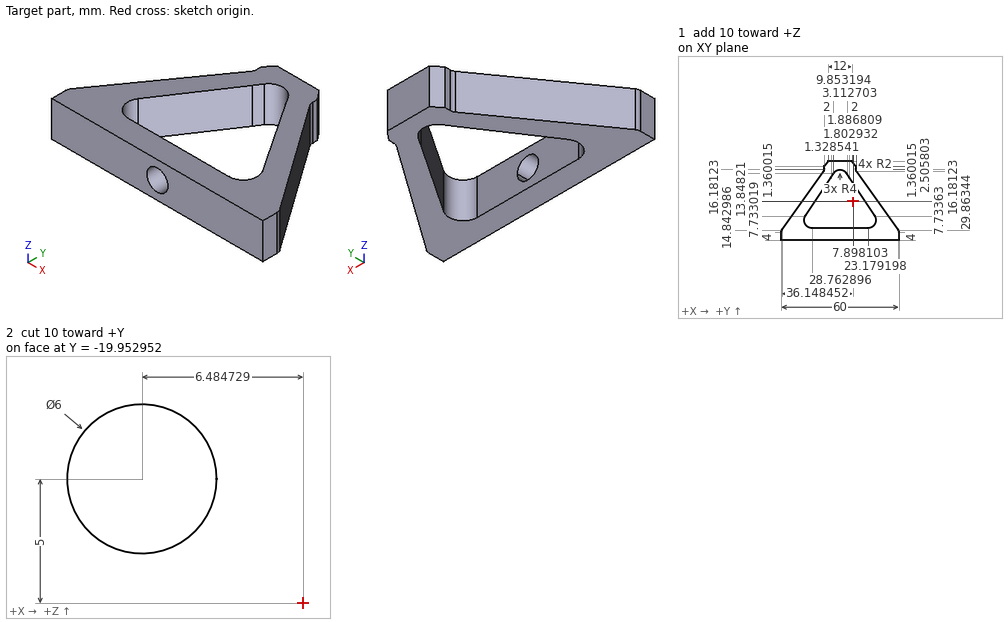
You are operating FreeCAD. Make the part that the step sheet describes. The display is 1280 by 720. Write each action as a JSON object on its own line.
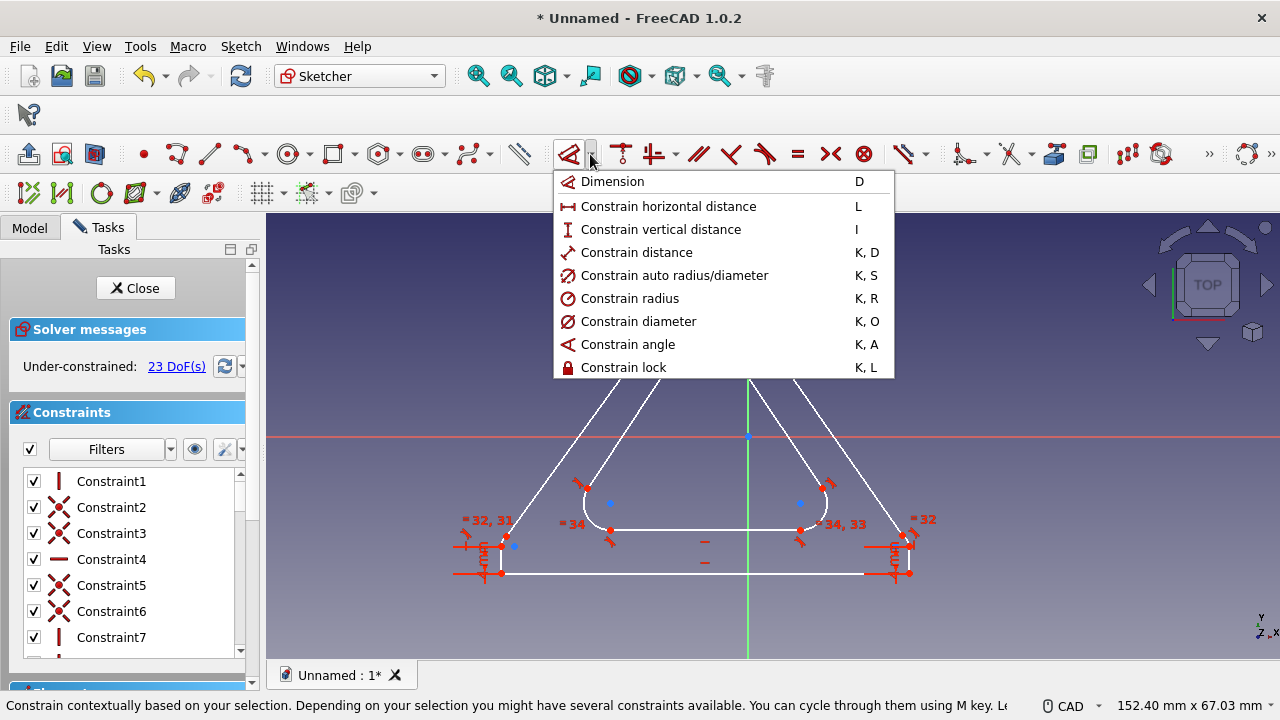
{"action": "left_click", "coordinate": [724, 206]}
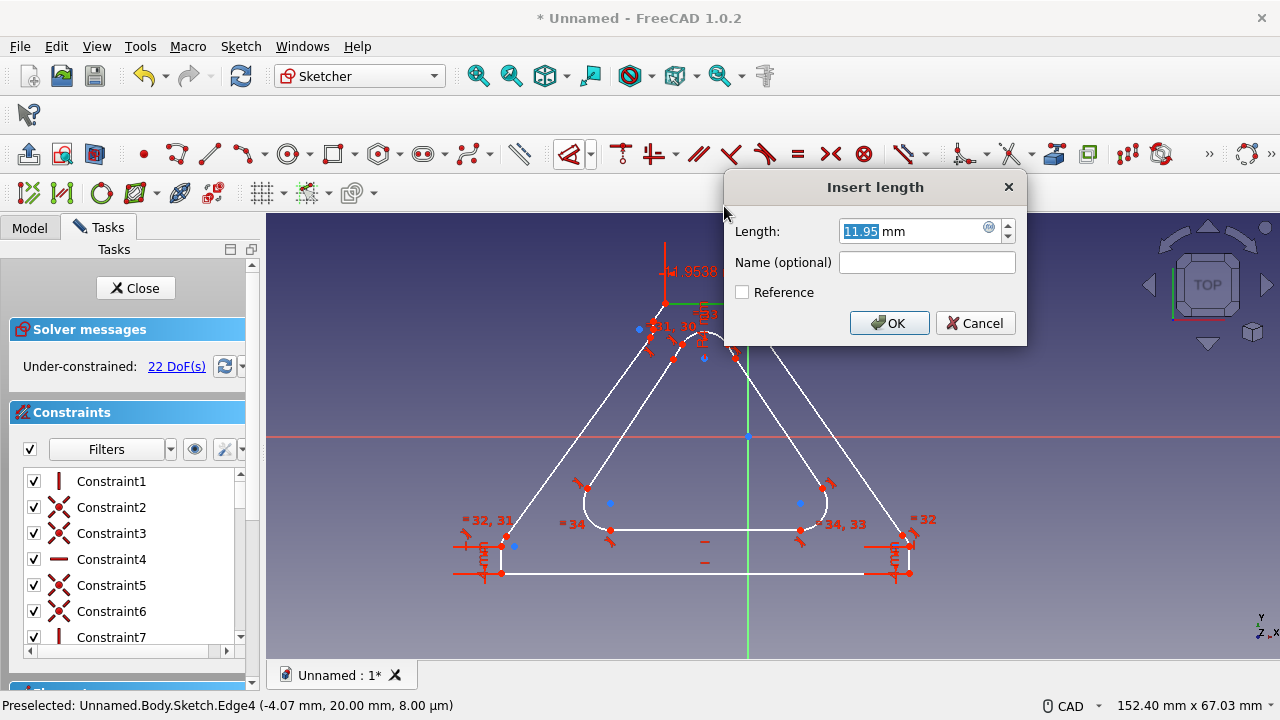
{"action": "type", "text": "12"}
{"action": "key", "text": "Return"}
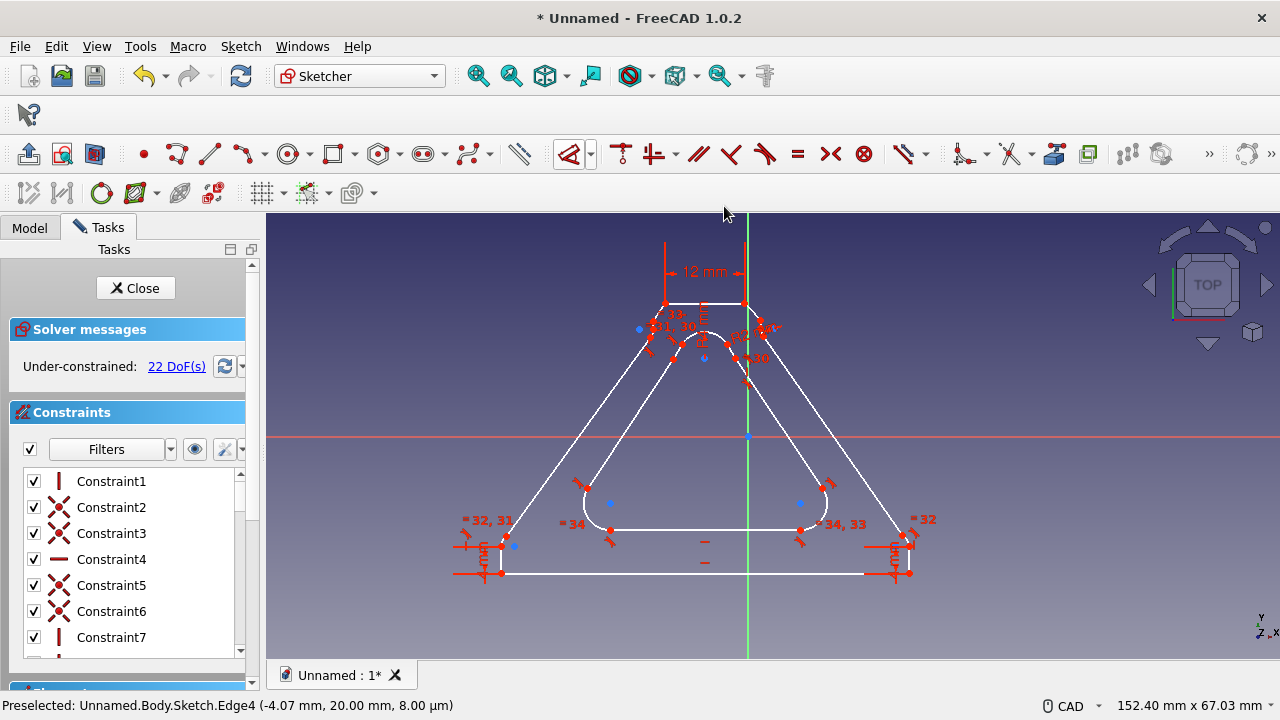
{"action": "left_click", "coordinate": [624, 574]}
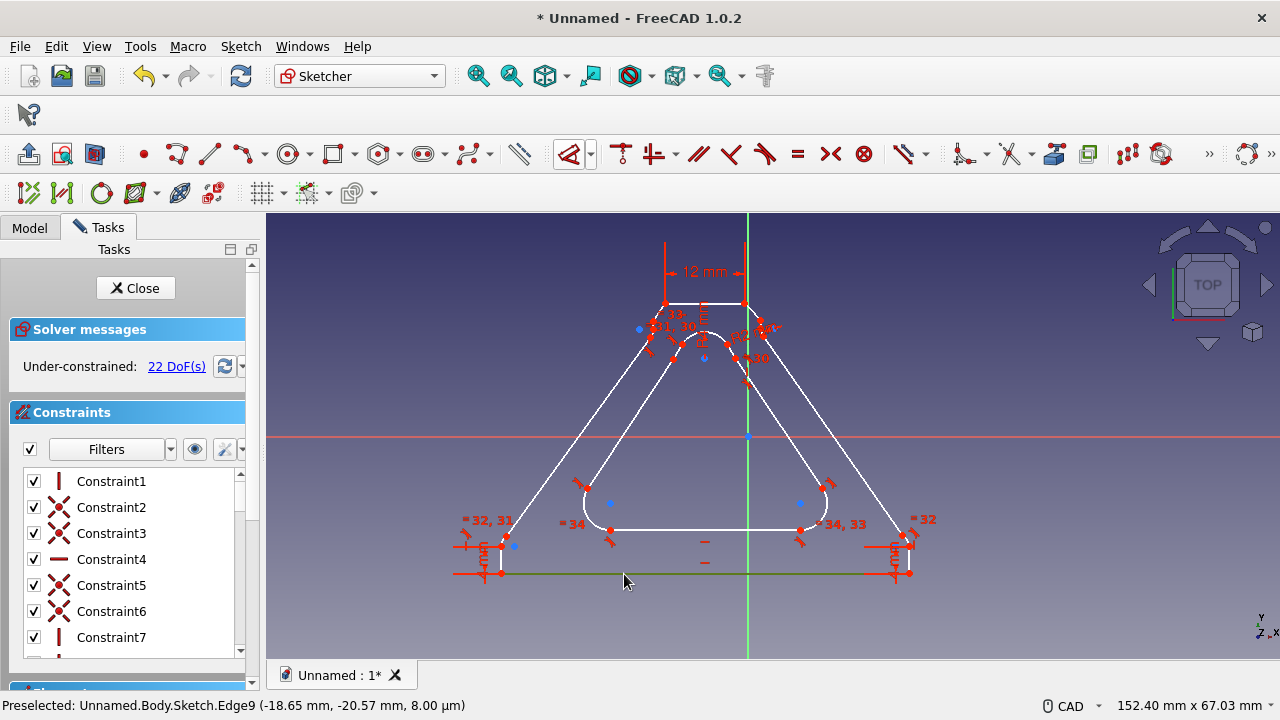
{"action": "key", "text": "l"}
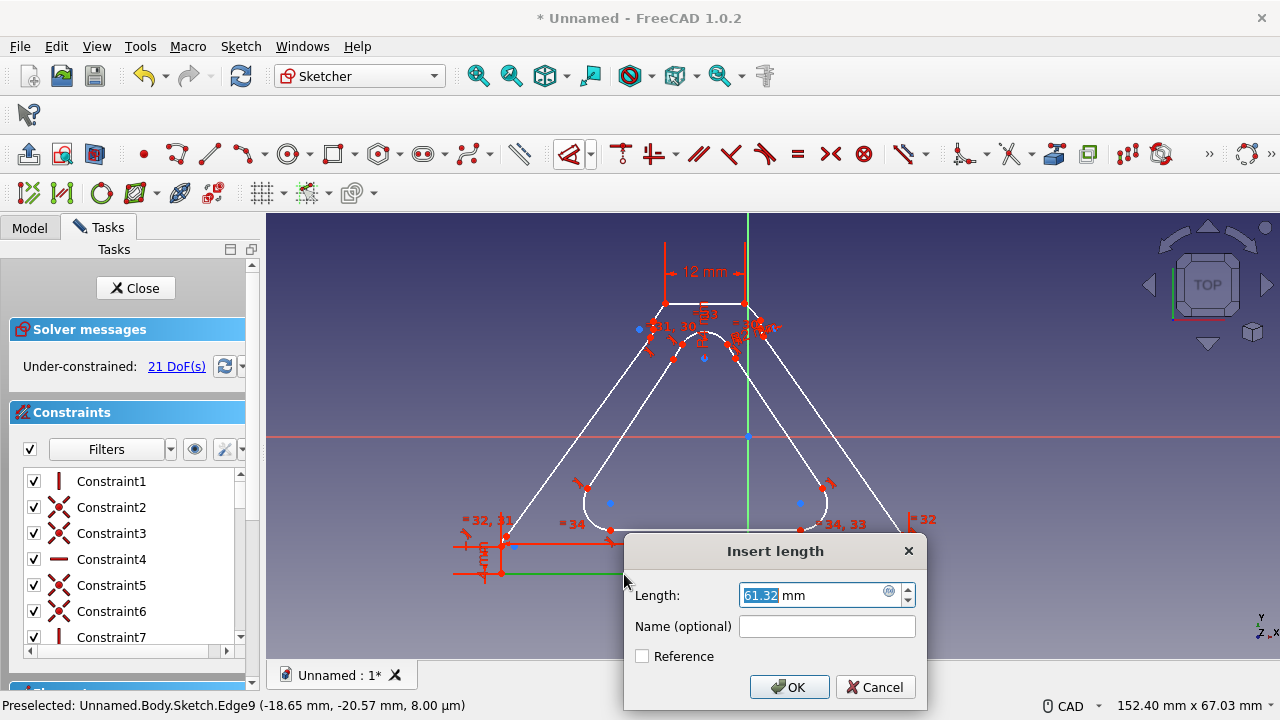
{"action": "type", "text": "60"}
{"action": "key", "text": "Return"}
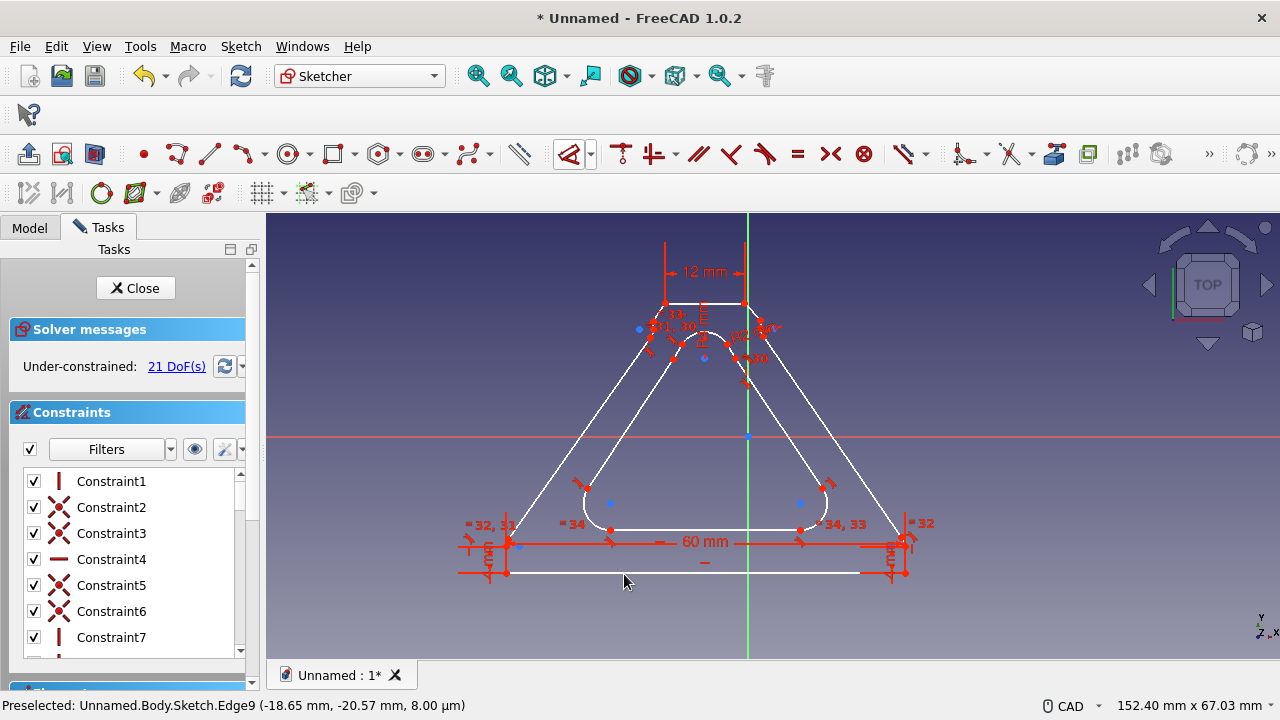
{"action": "scroll", "coordinate": [751, 310], "scroll_direction": "up", "scroll_amount": 6}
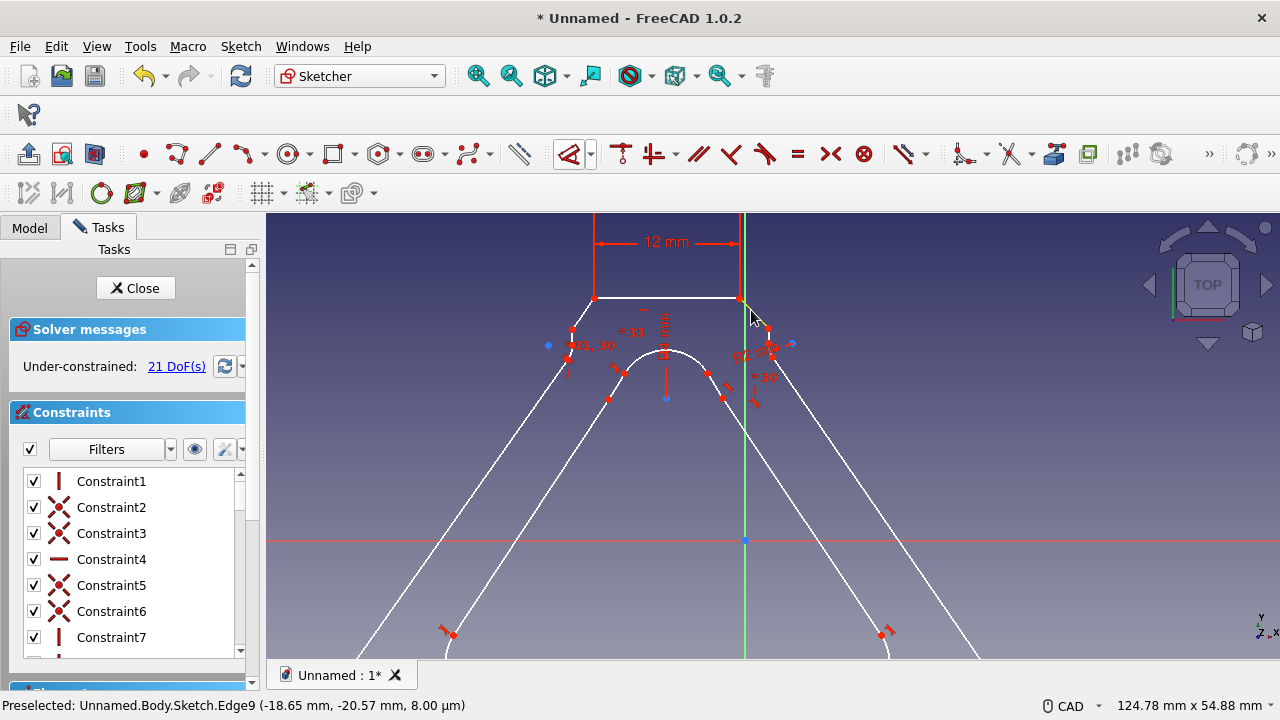
{"action": "left_click", "coordinate": [751, 310]}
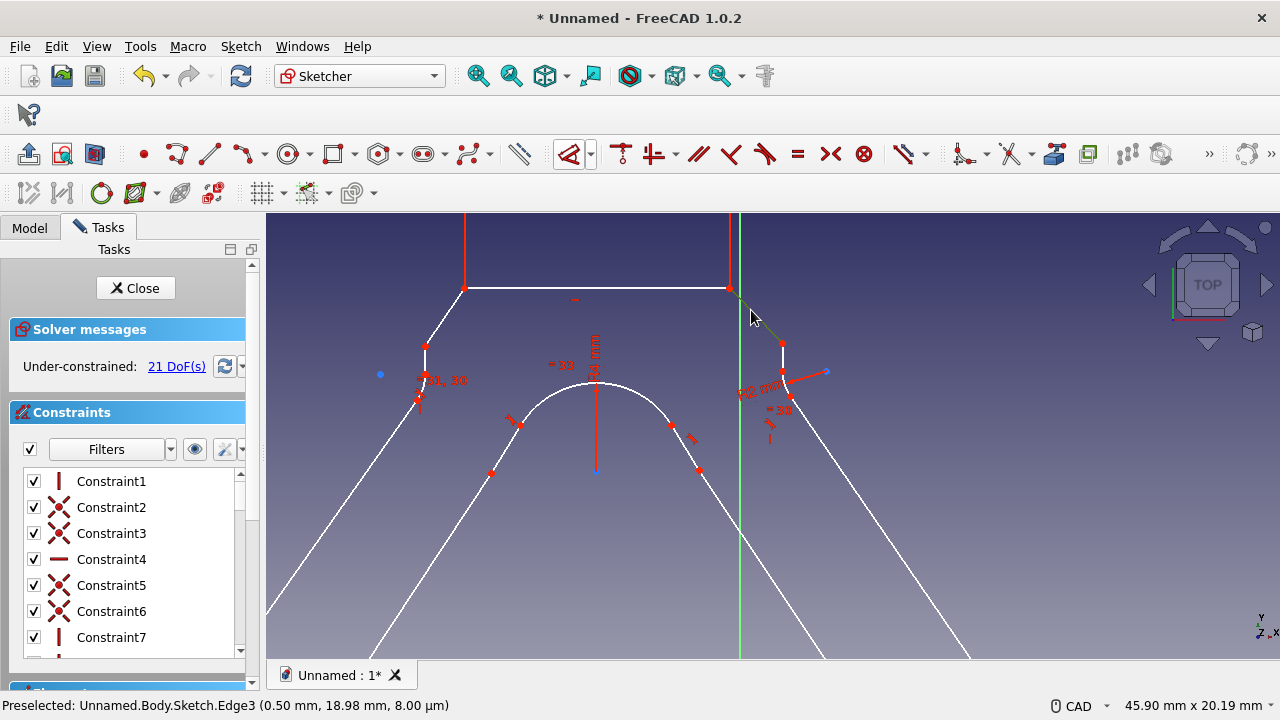
{"action": "left_click", "coordinate": [590, 154]}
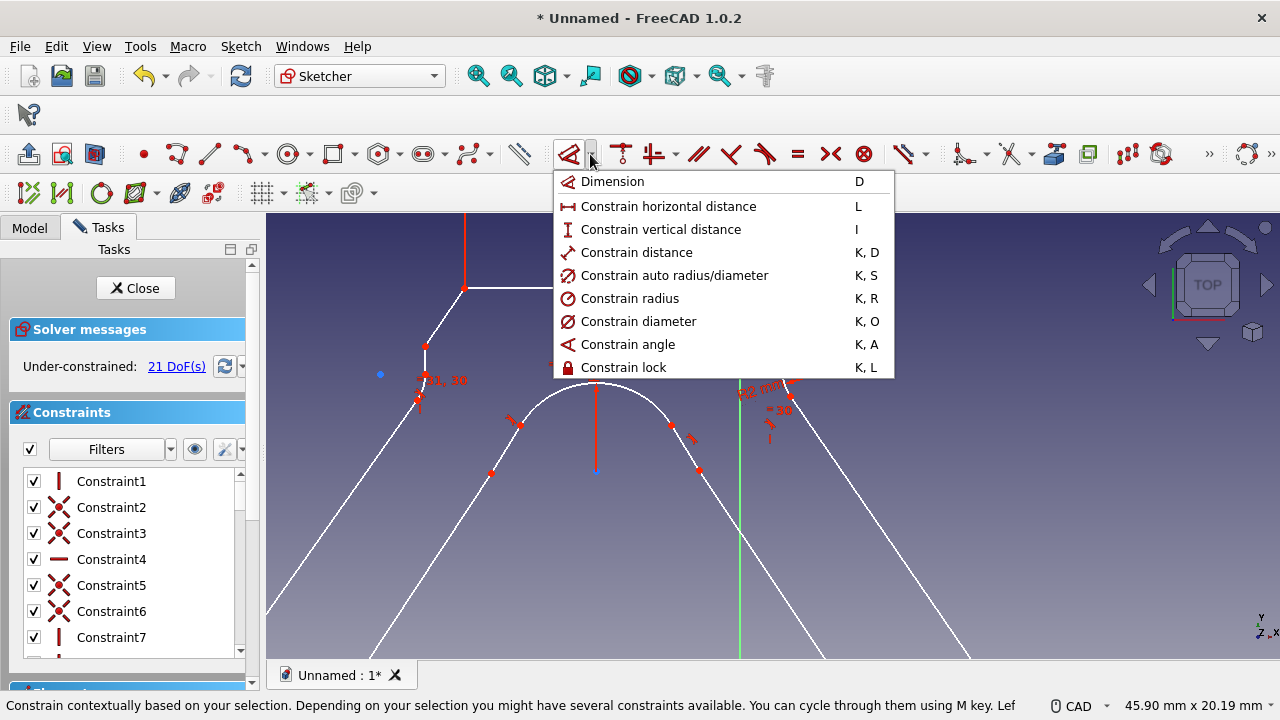
{"action": "left_click", "coordinate": [724, 206]}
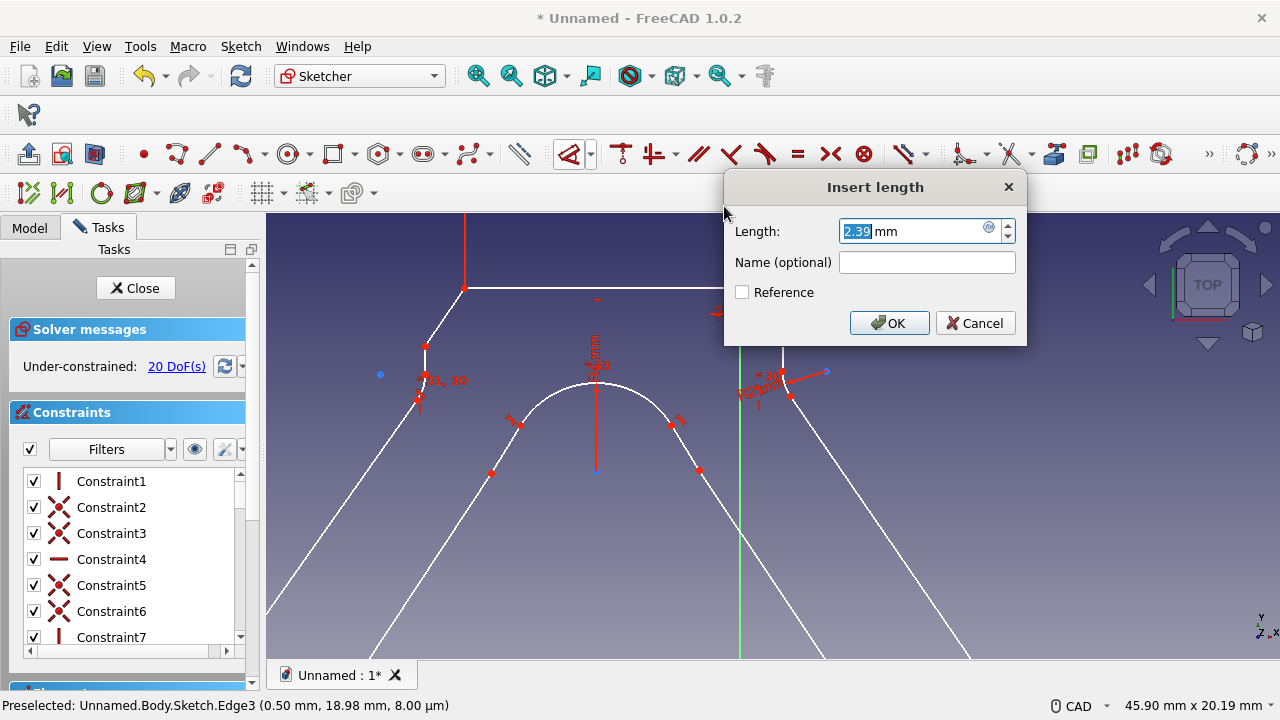
{"action": "type", "text": "2"}
{"action": "key", "text": "Return"}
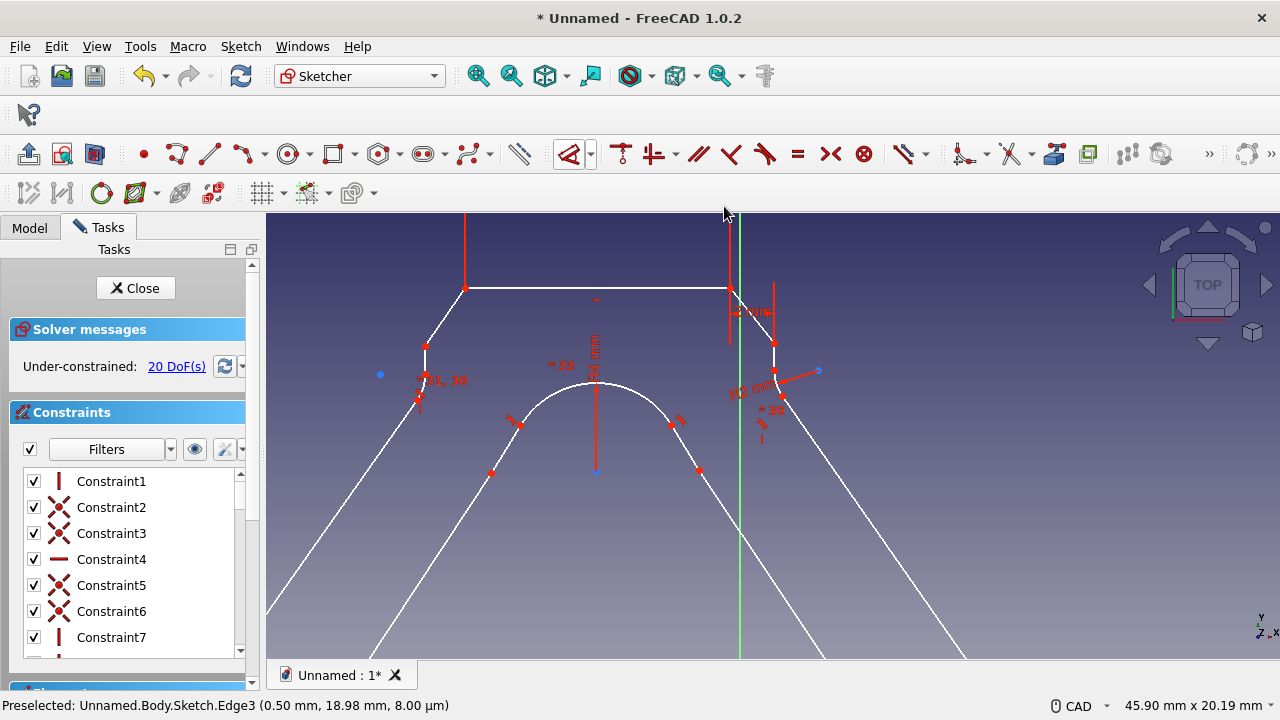
{"action": "left_click", "coordinate": [453, 306]}